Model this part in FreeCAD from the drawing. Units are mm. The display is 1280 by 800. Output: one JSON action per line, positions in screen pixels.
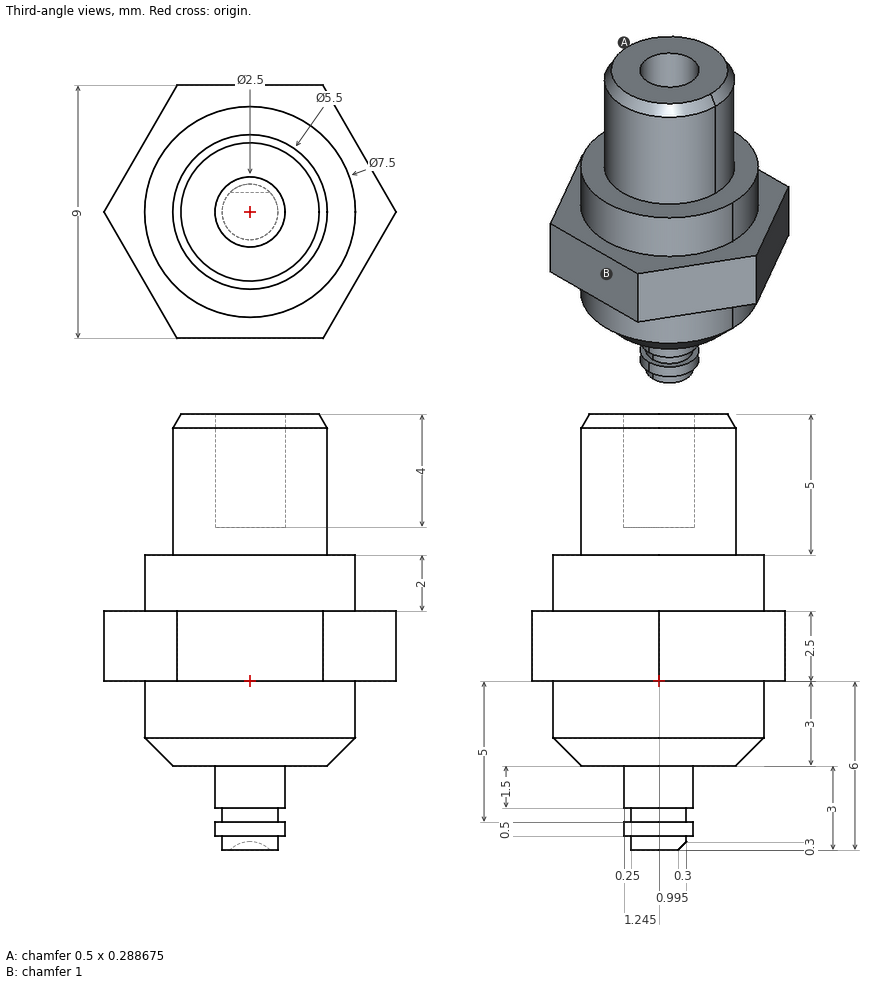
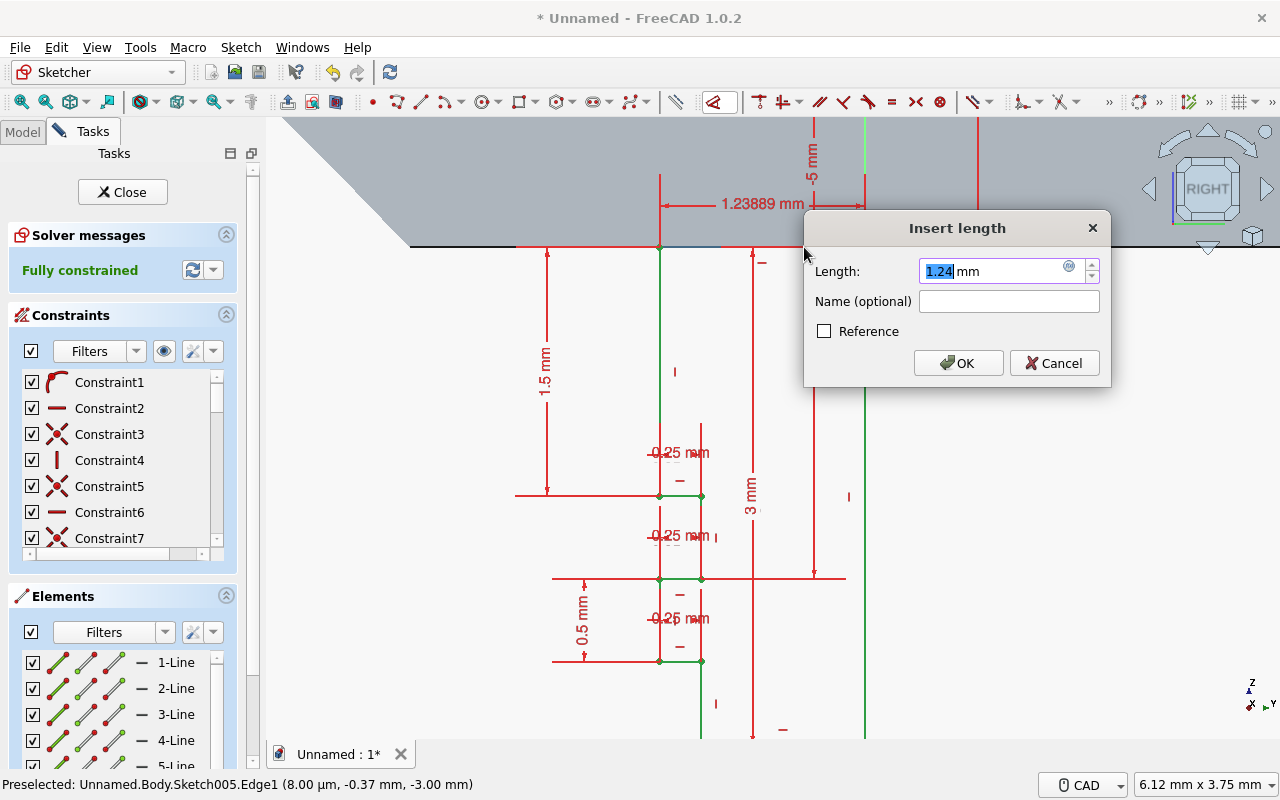
{"action": "type", "text": "1.245"}
{"action": "key", "text": "Return"}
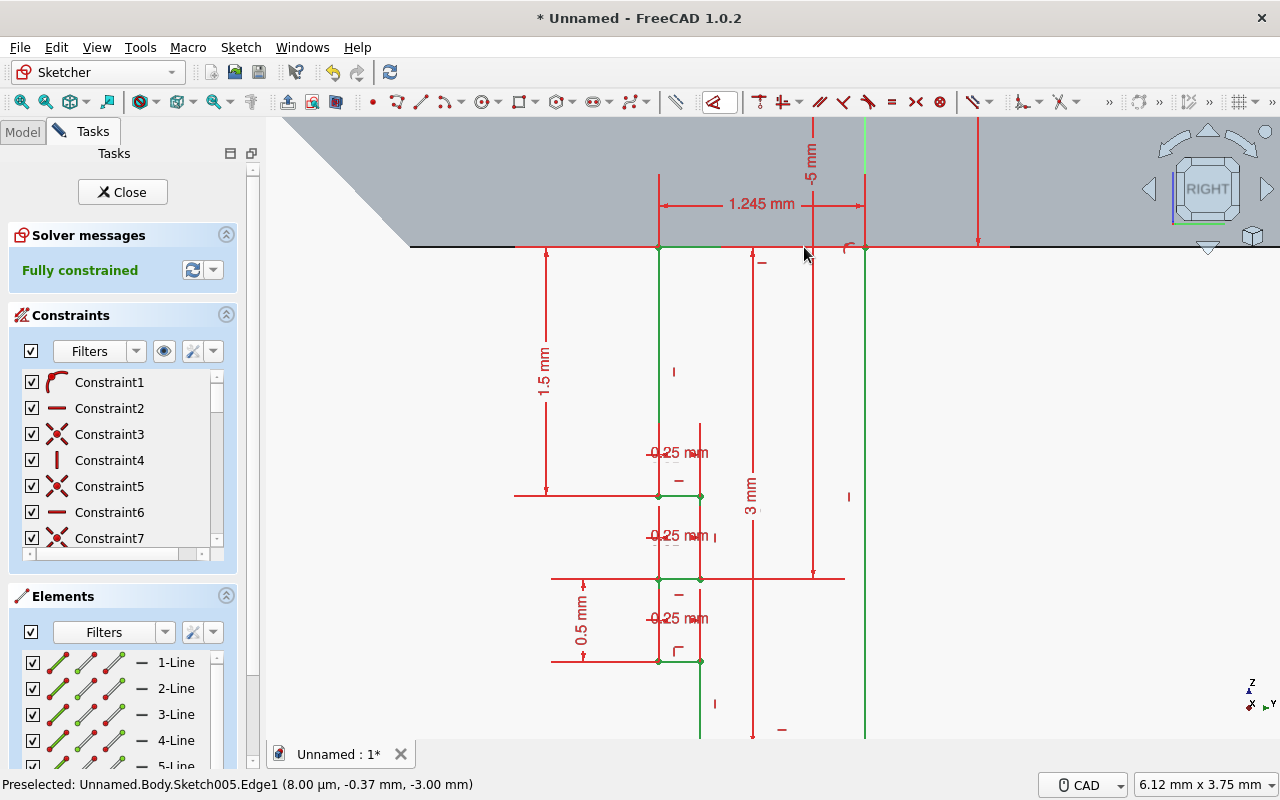
{"action": "left_click", "coordinate": [123, 192]}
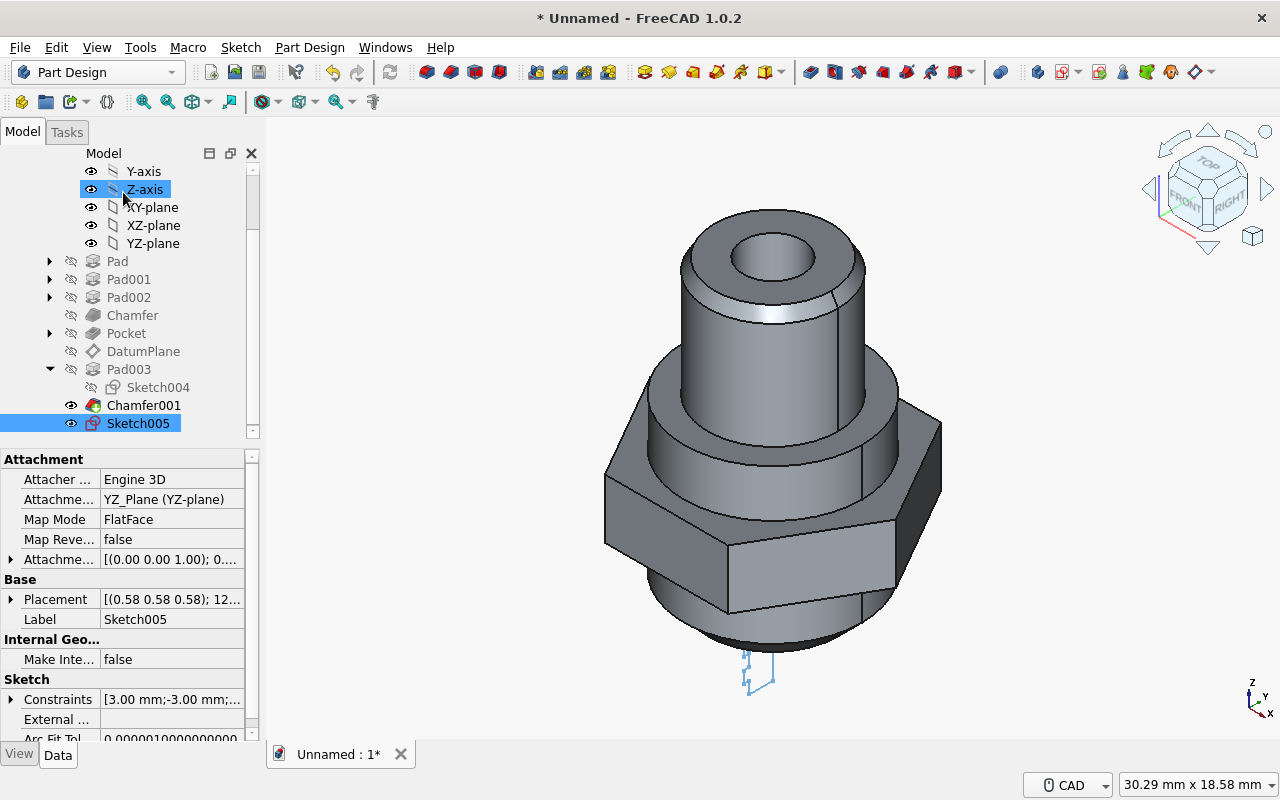
{"action": "left_click", "coordinate": [670, 72]}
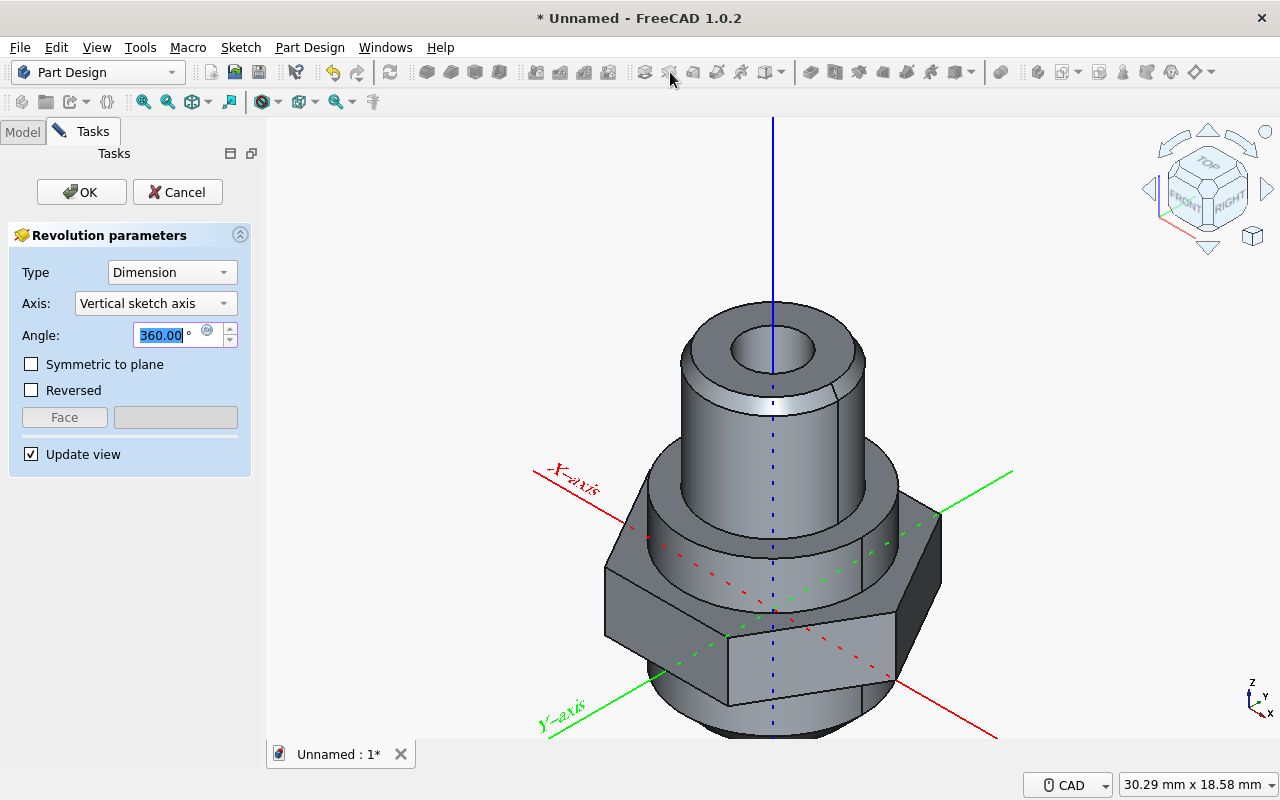
{"action": "left_click", "coordinate": [82, 192]}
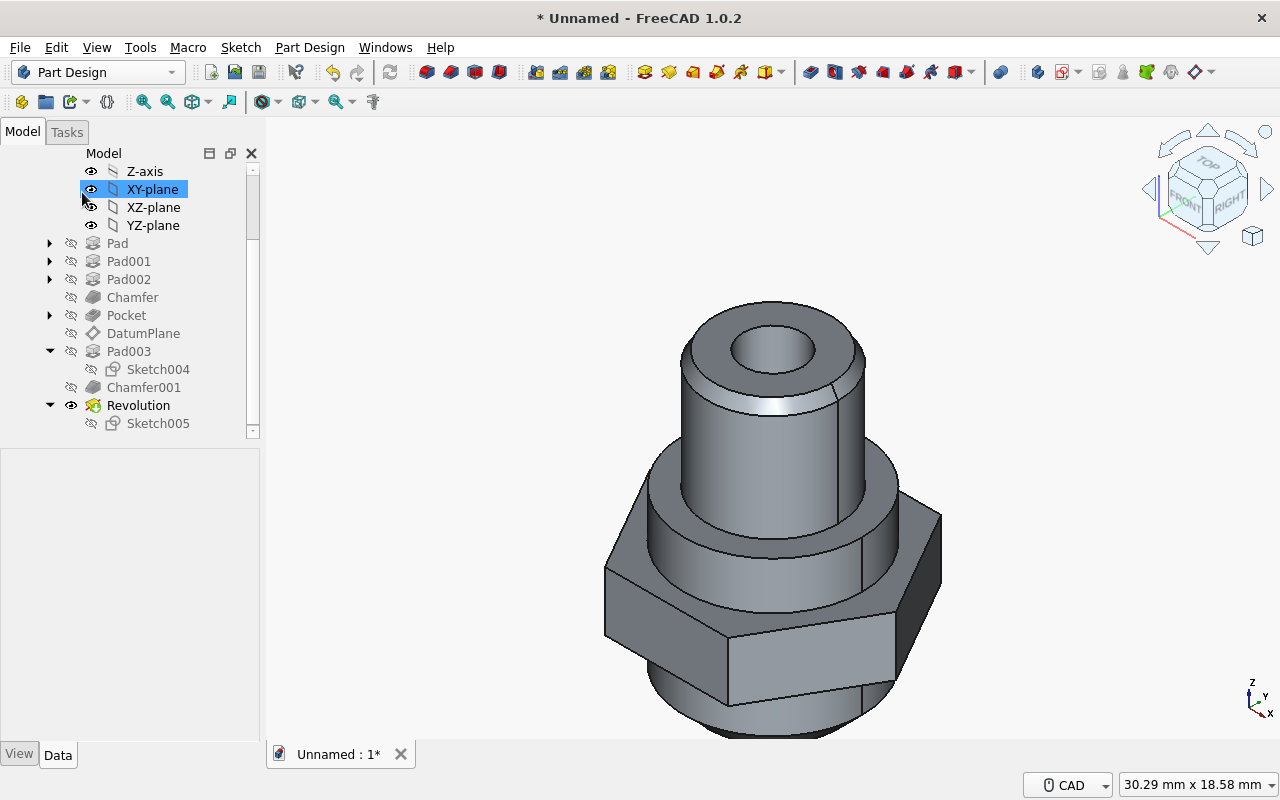
{"action": "left_click", "coordinate": [144, 102]}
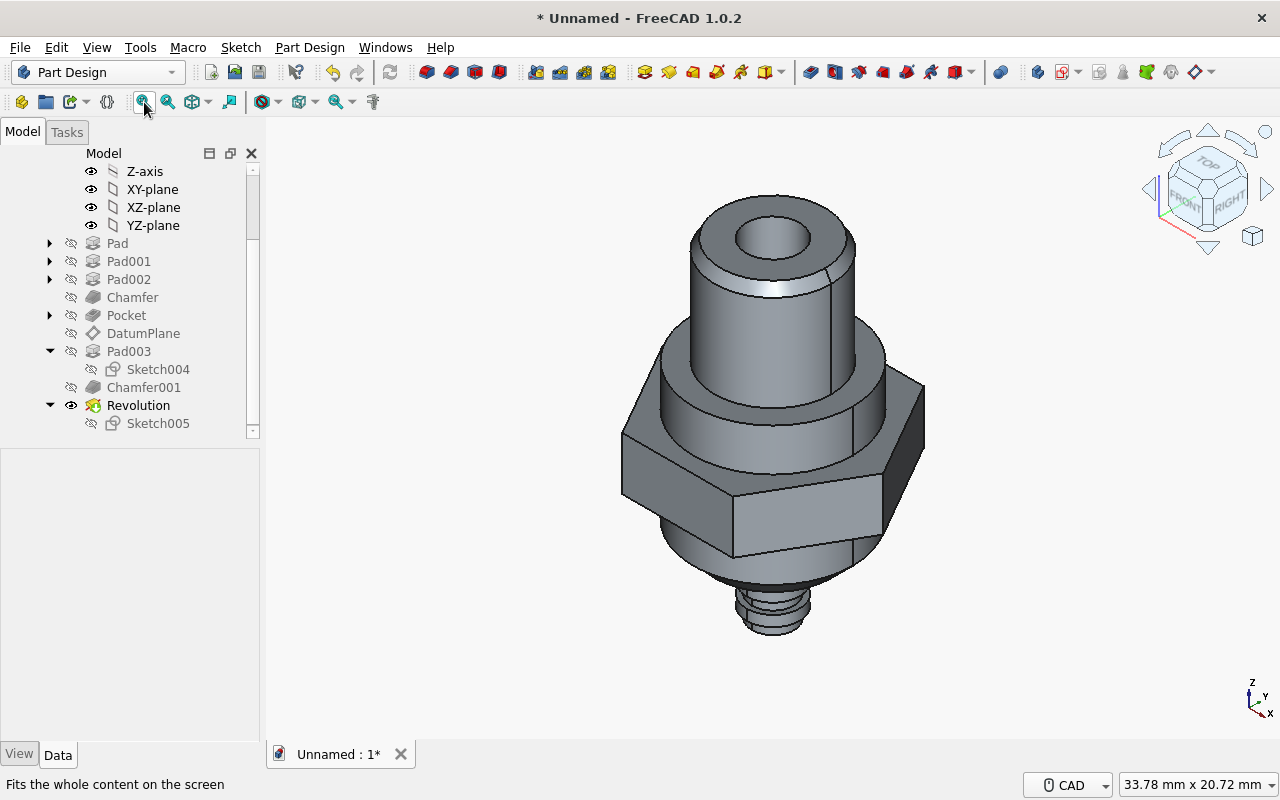
{"action": "left_click", "coordinate": [1062, 72]}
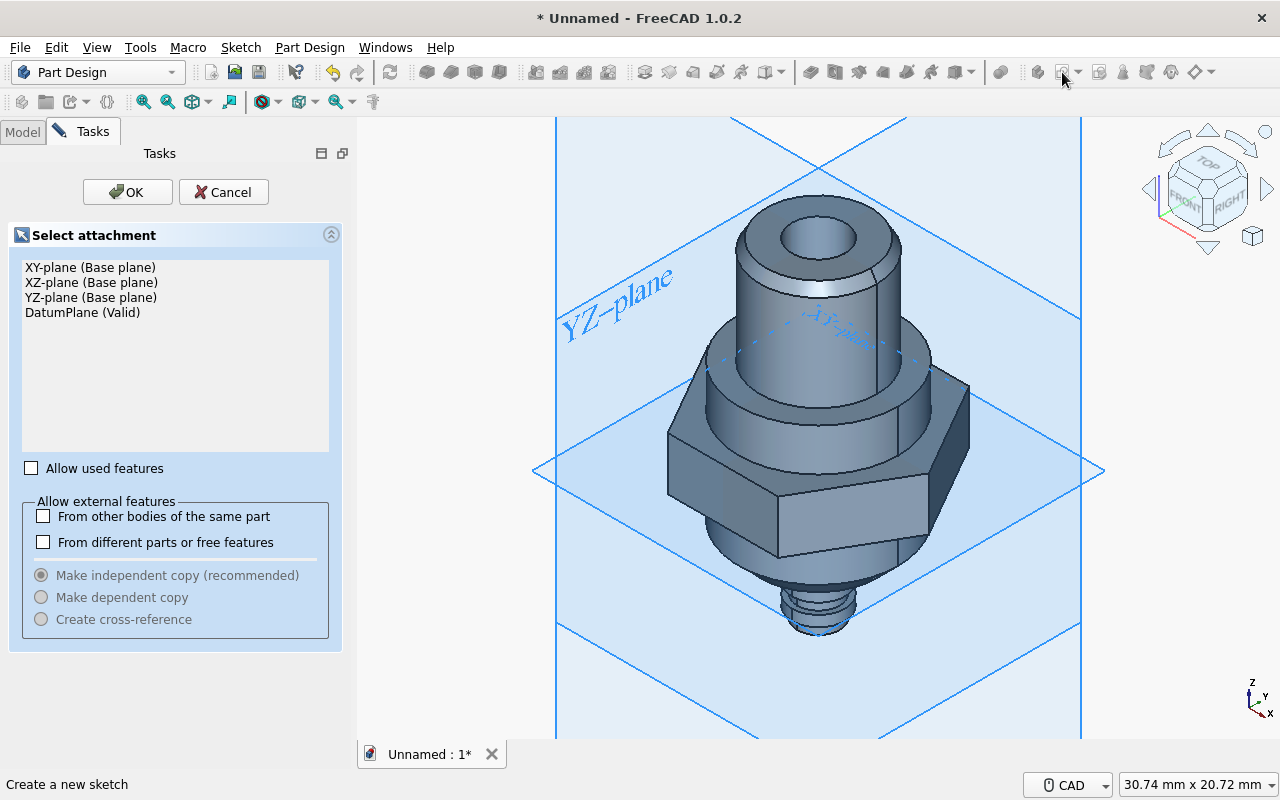
{"action": "left_click", "coordinate": [82, 298]}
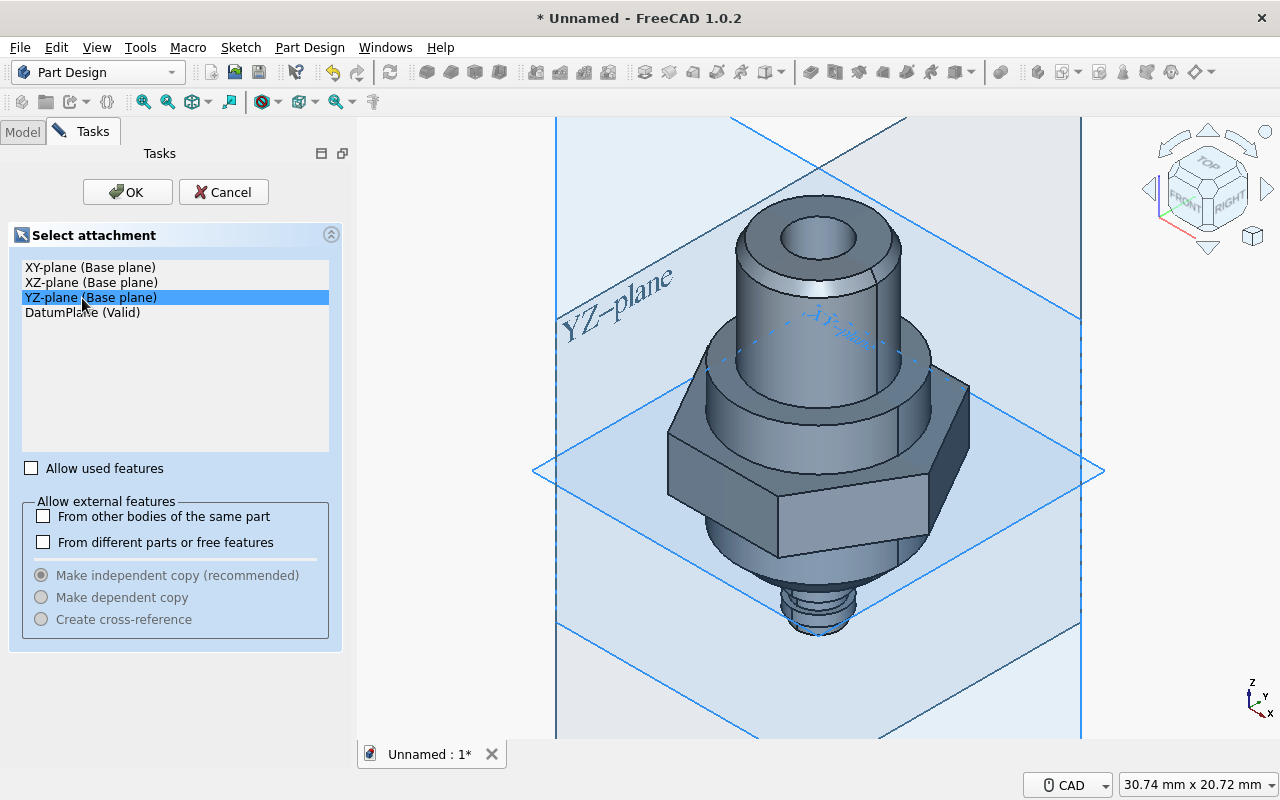
{"action": "left_click", "coordinate": [128, 192]}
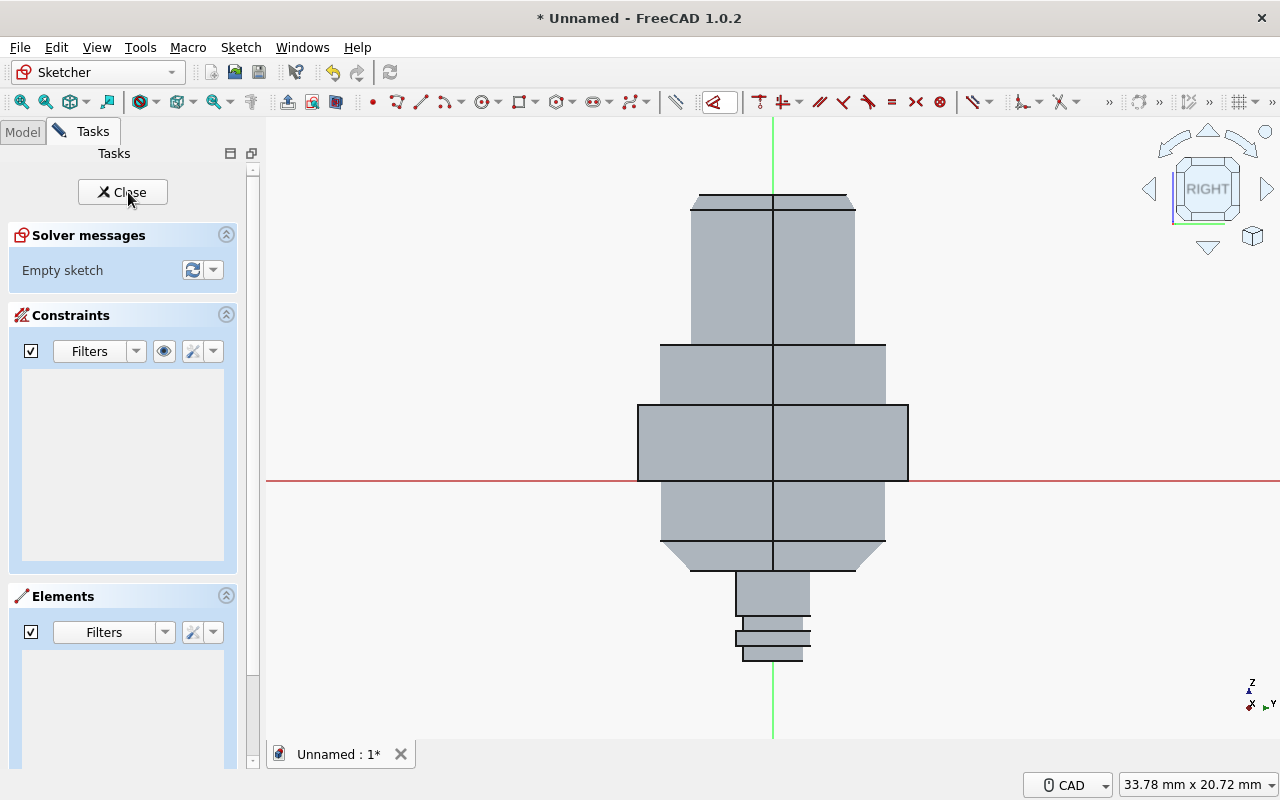
{"action": "key", "text": "q s"}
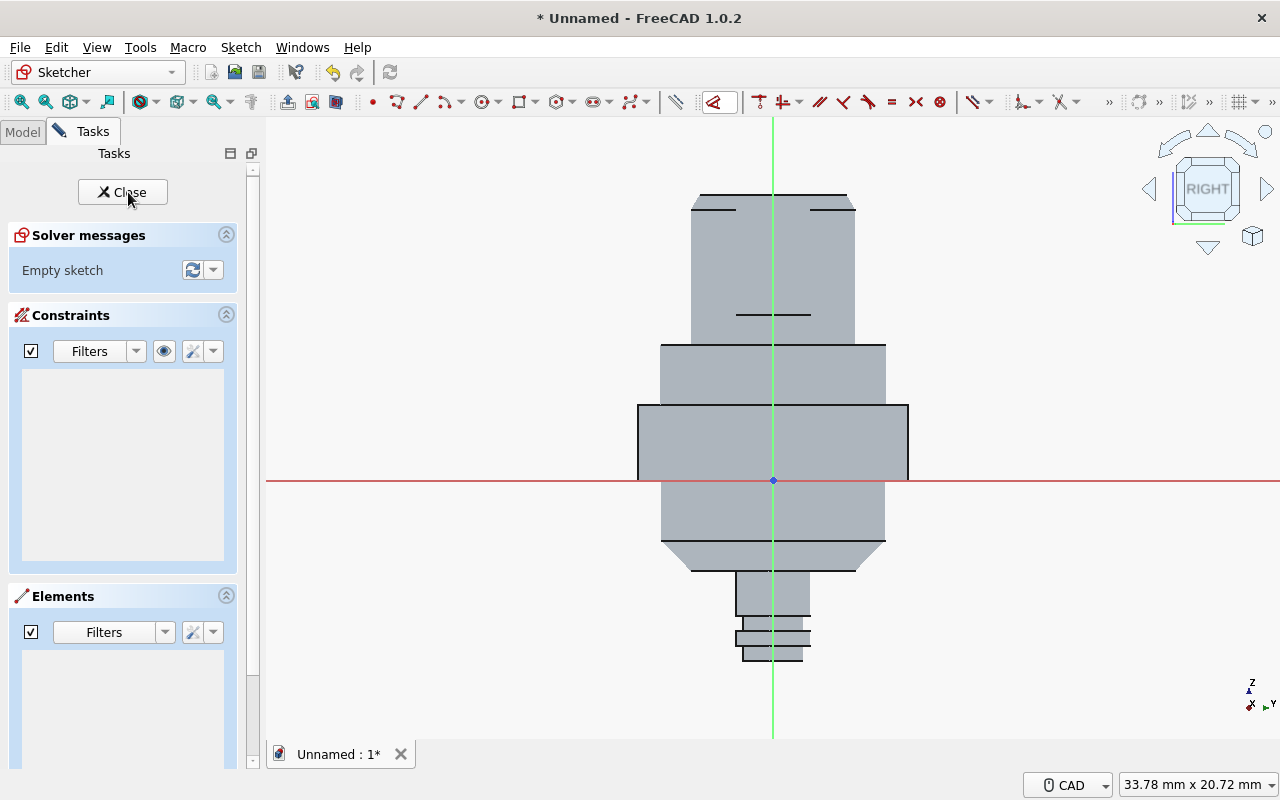
{"action": "scroll", "coordinate": [803, 668], "scroll_direction": "up", "scroll_amount": 15}